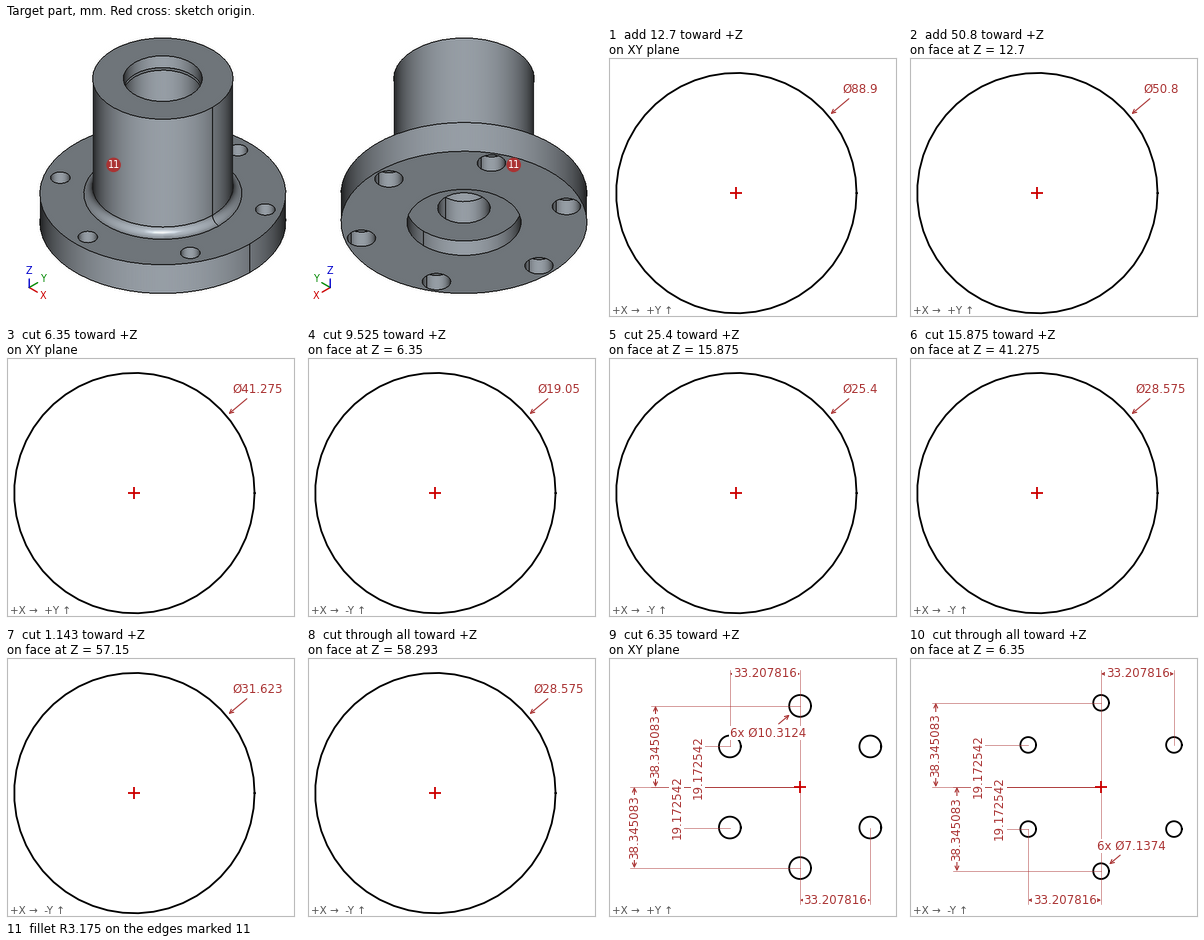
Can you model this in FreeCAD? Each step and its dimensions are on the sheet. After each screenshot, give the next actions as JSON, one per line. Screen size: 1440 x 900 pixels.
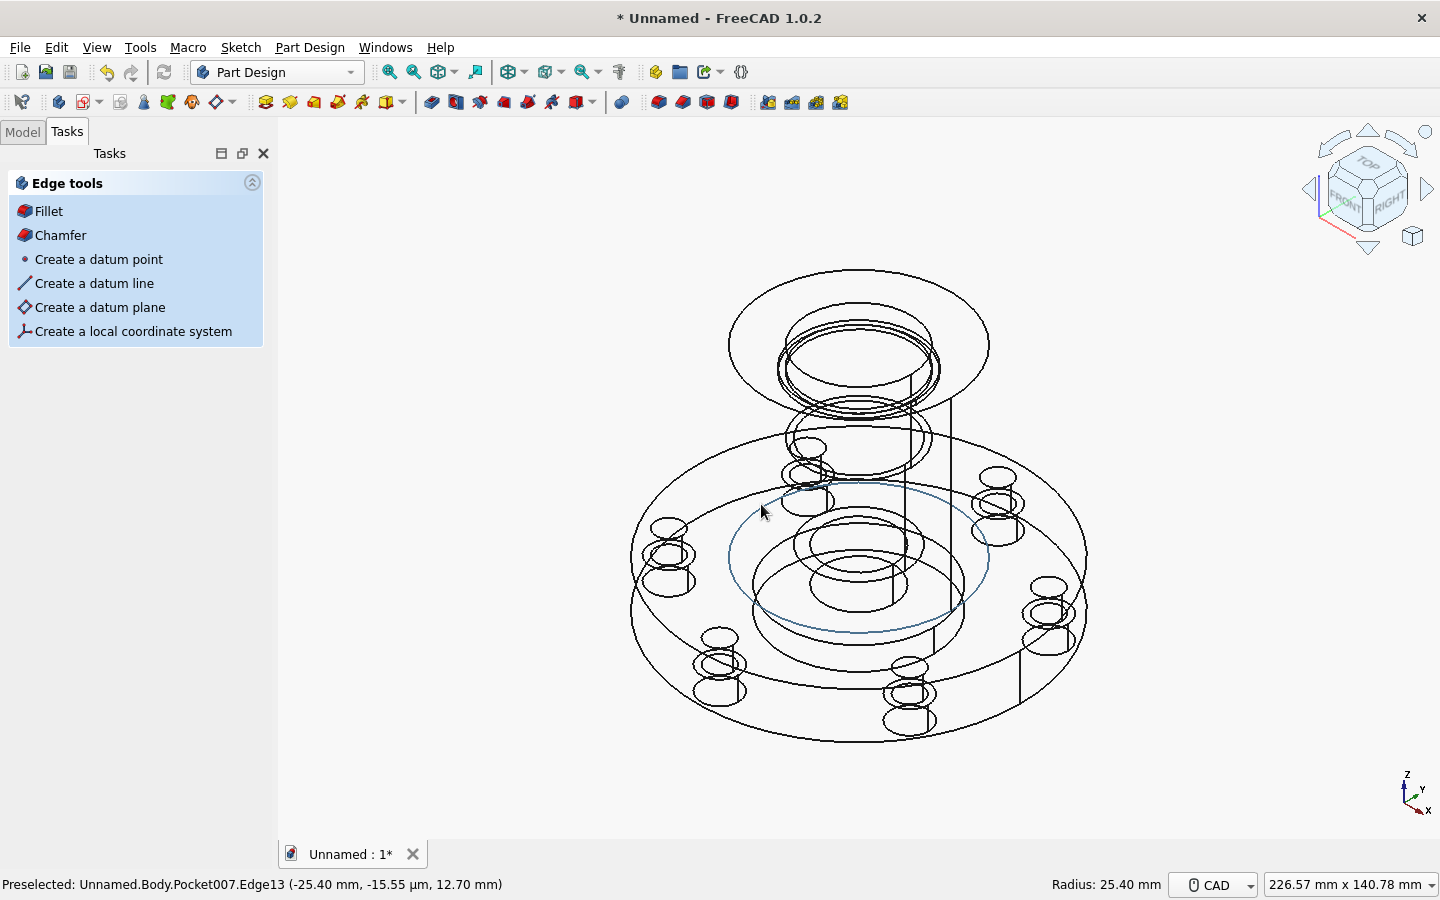
{"action": "key", "text": "v 1"}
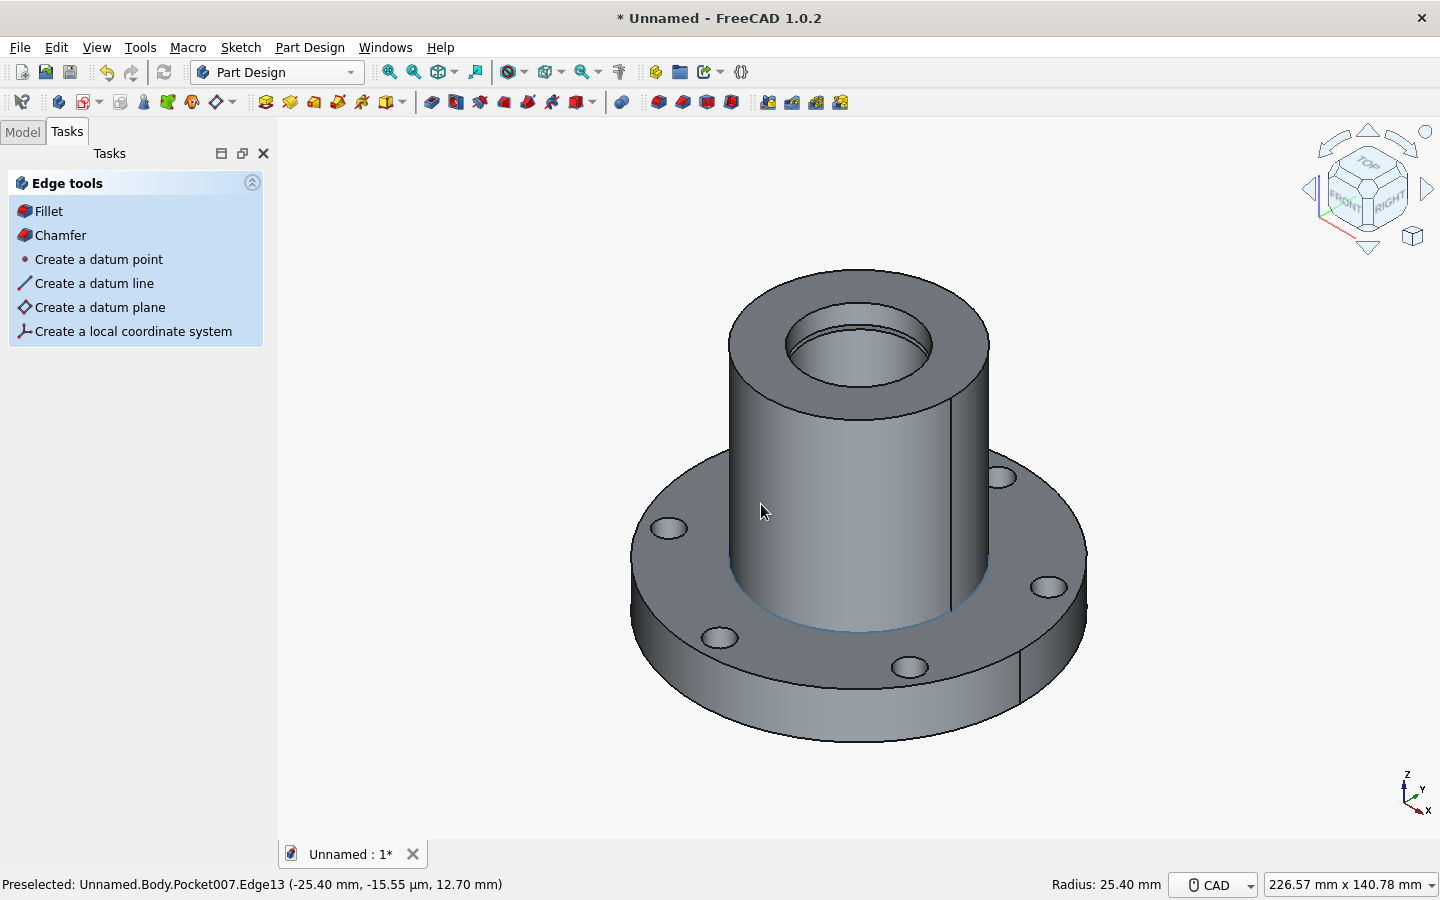
{"action": "left_click", "coordinate": [660, 102]}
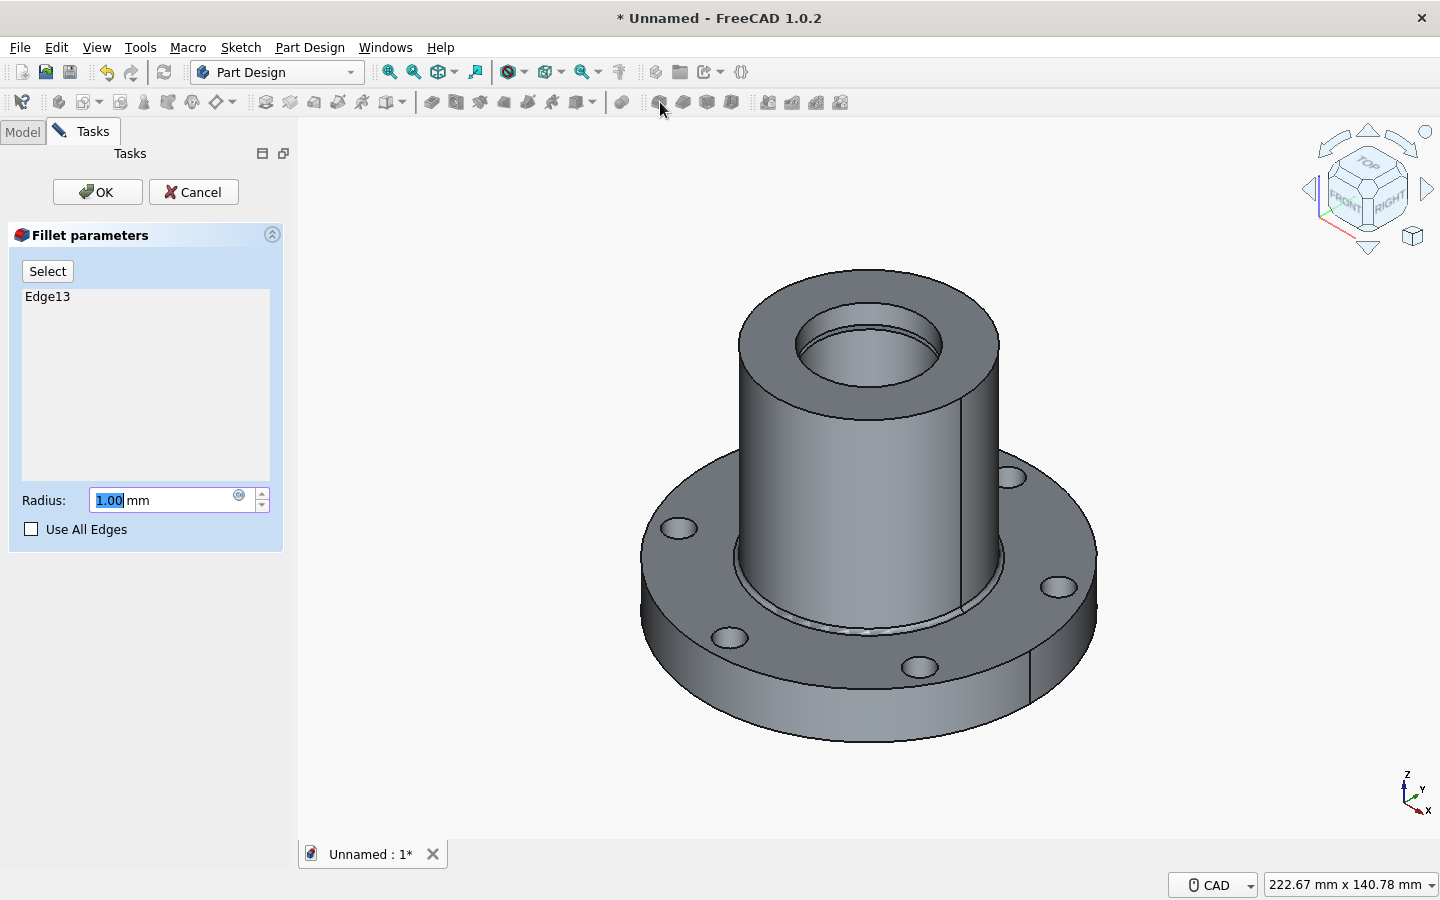
{"action": "type", "text": "3.175"}
{"action": "key", "text": "Tab"}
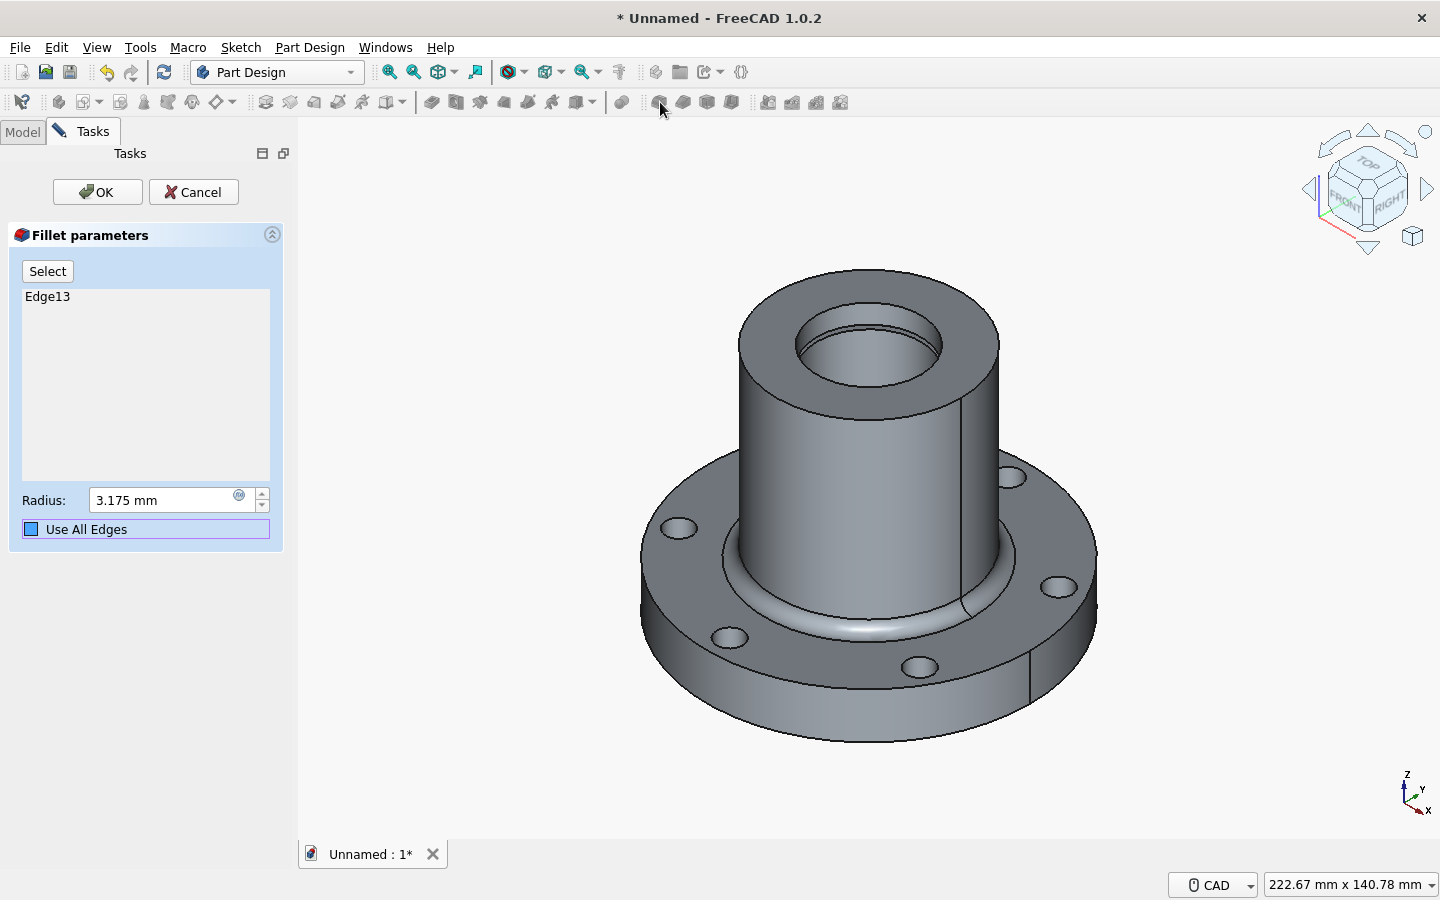
{"action": "left_click", "coordinate": [98, 192]}